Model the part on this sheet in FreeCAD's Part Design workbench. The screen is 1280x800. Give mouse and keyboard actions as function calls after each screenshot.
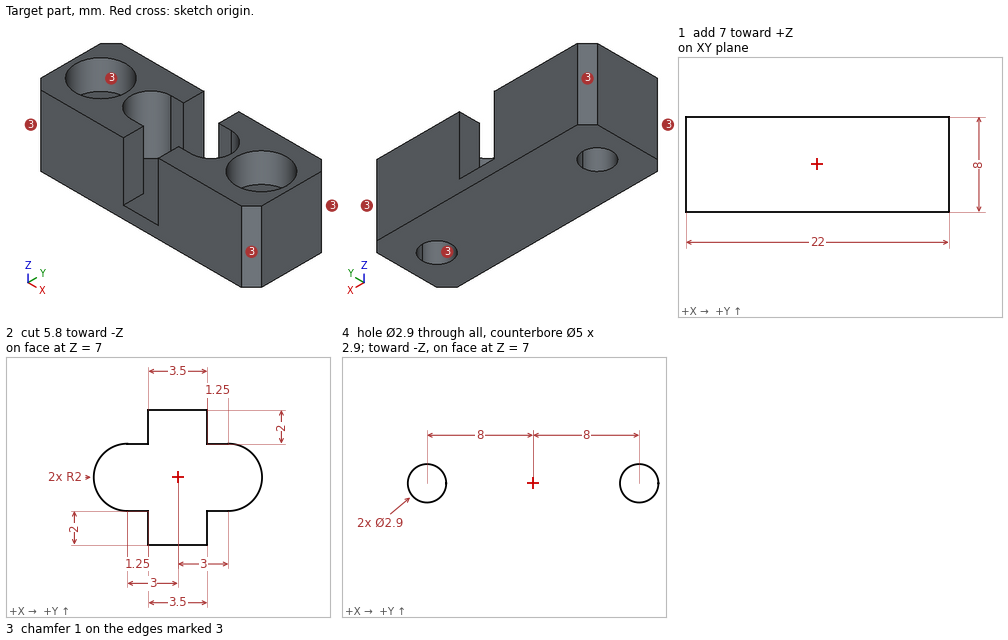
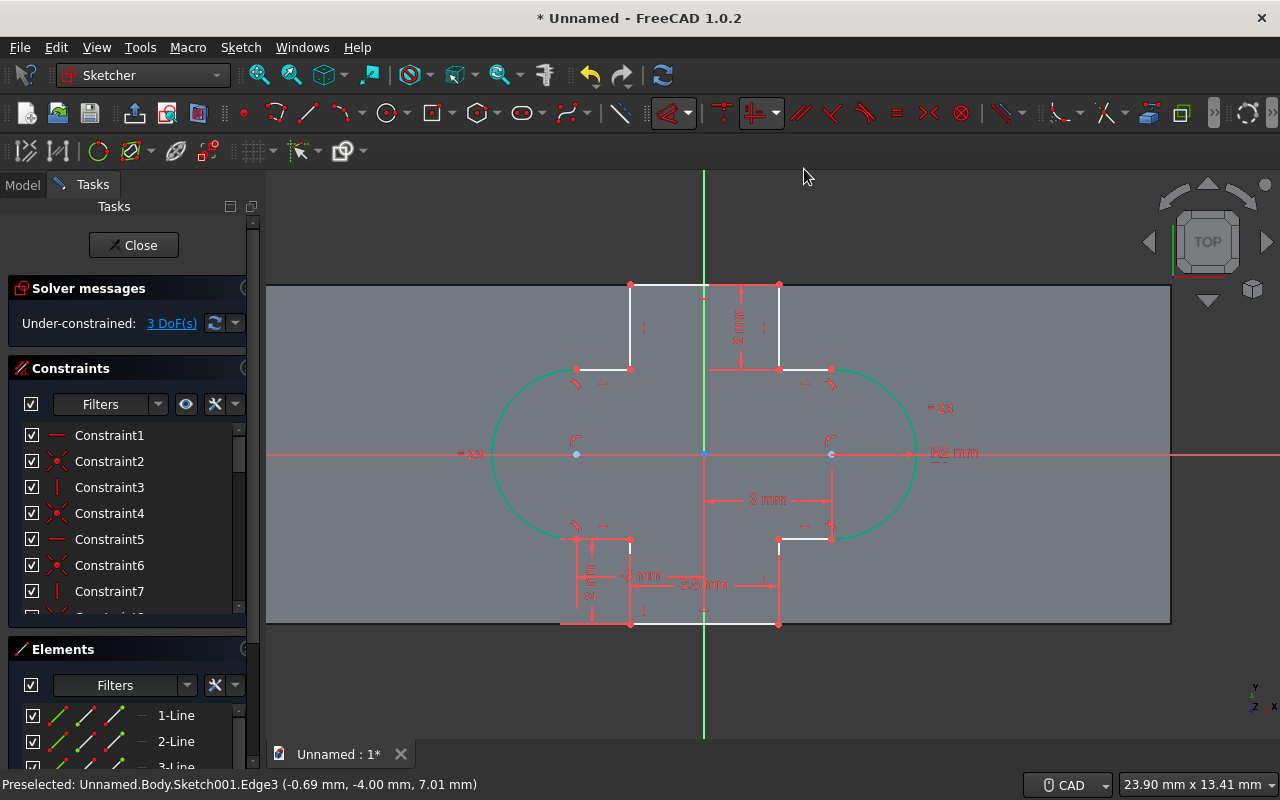
click(734, 285)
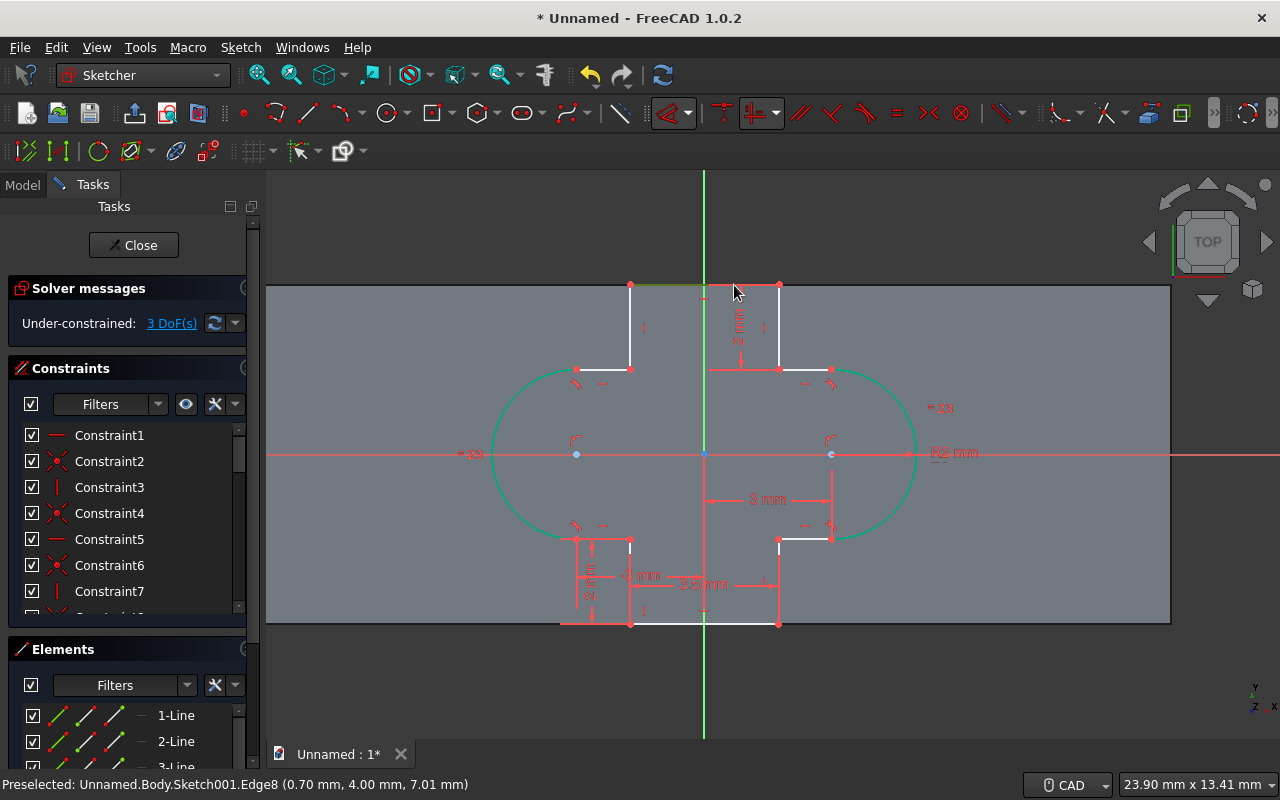
click(690, 114)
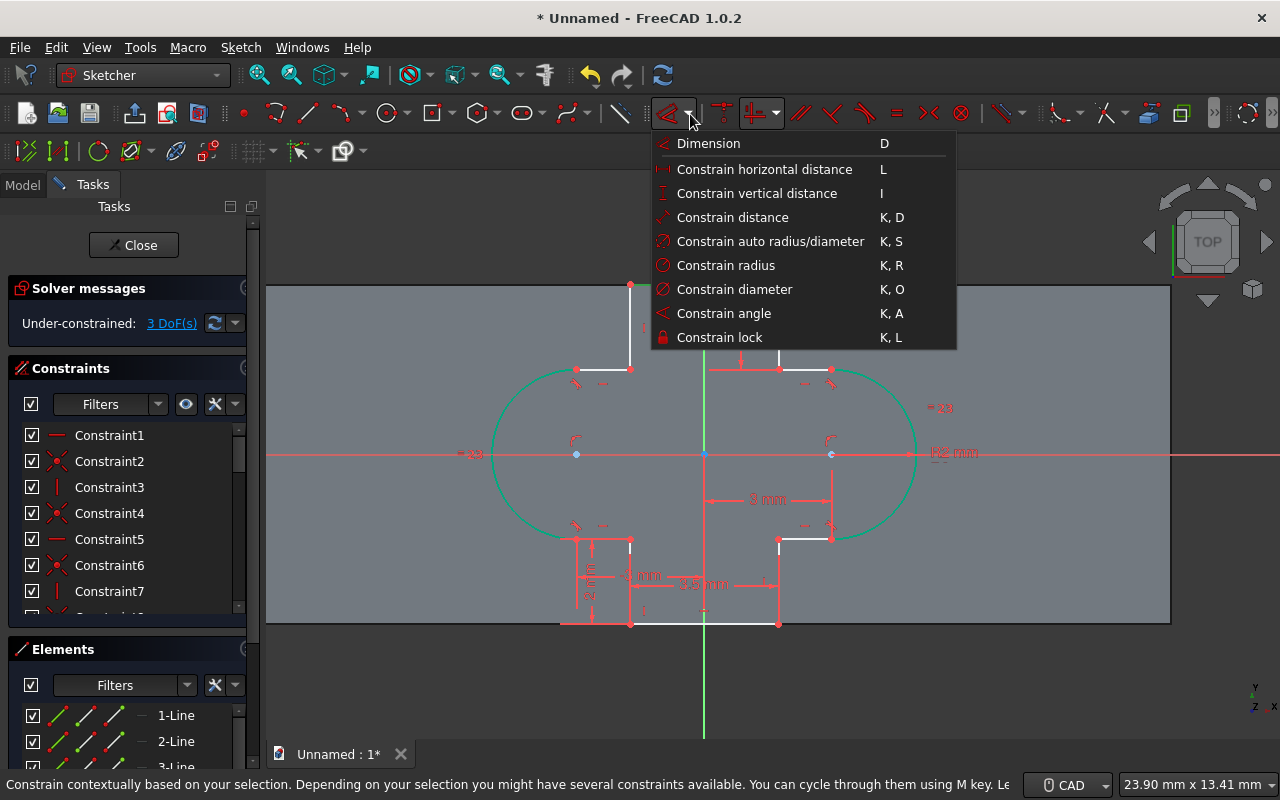
click(804, 169)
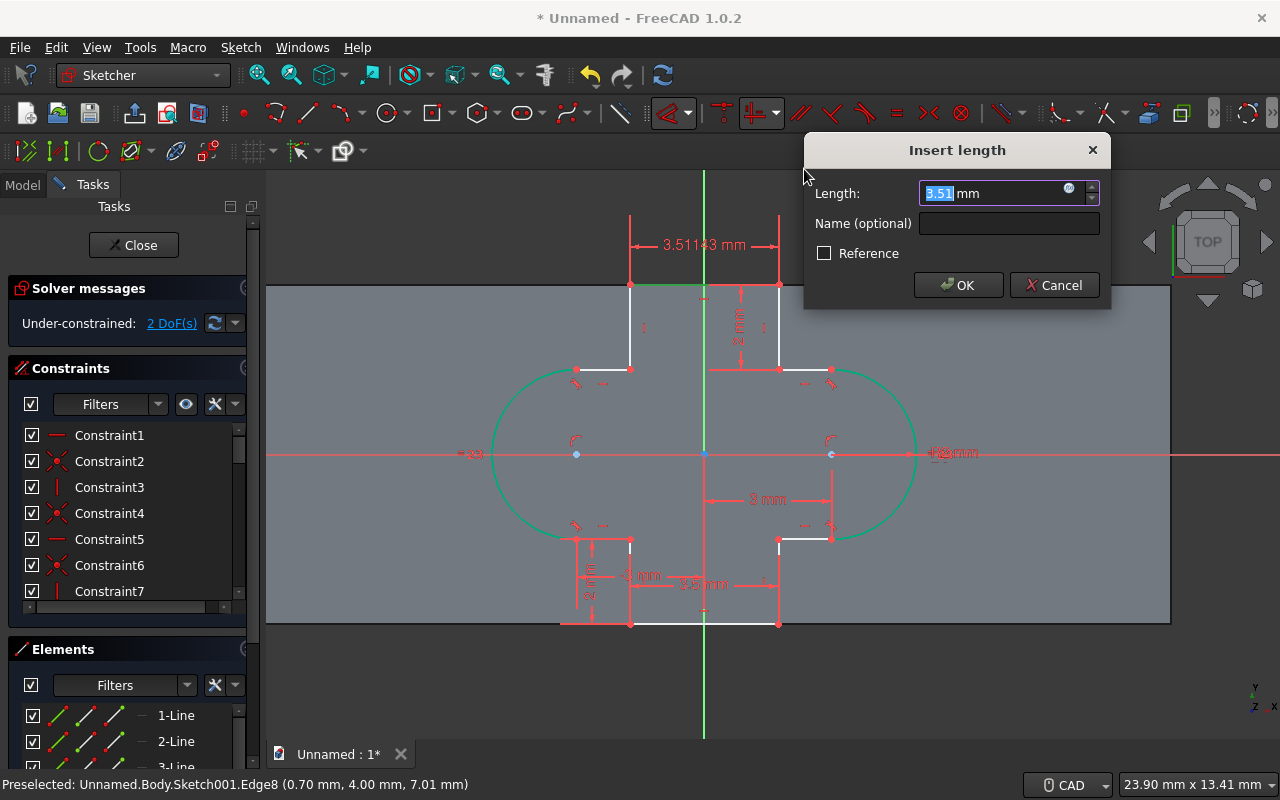
text(3.5)
key(Return)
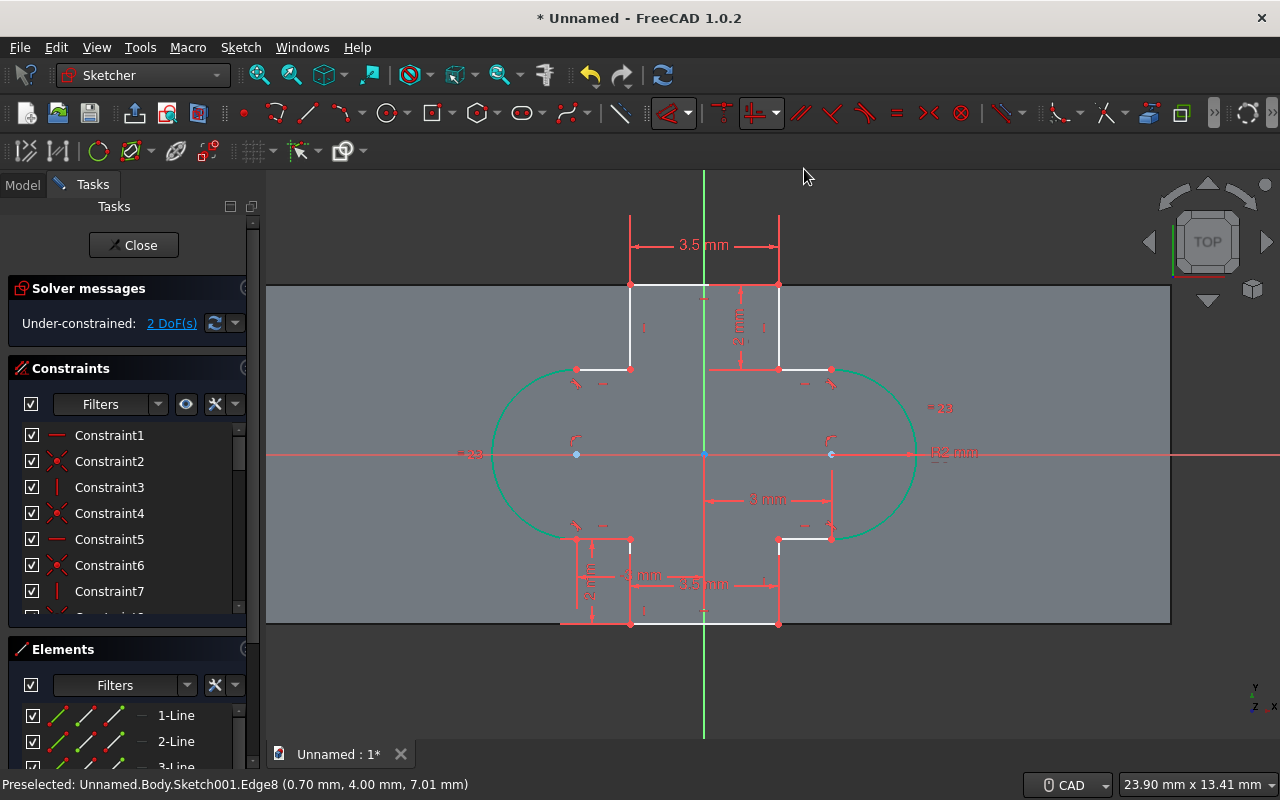
click(593, 539)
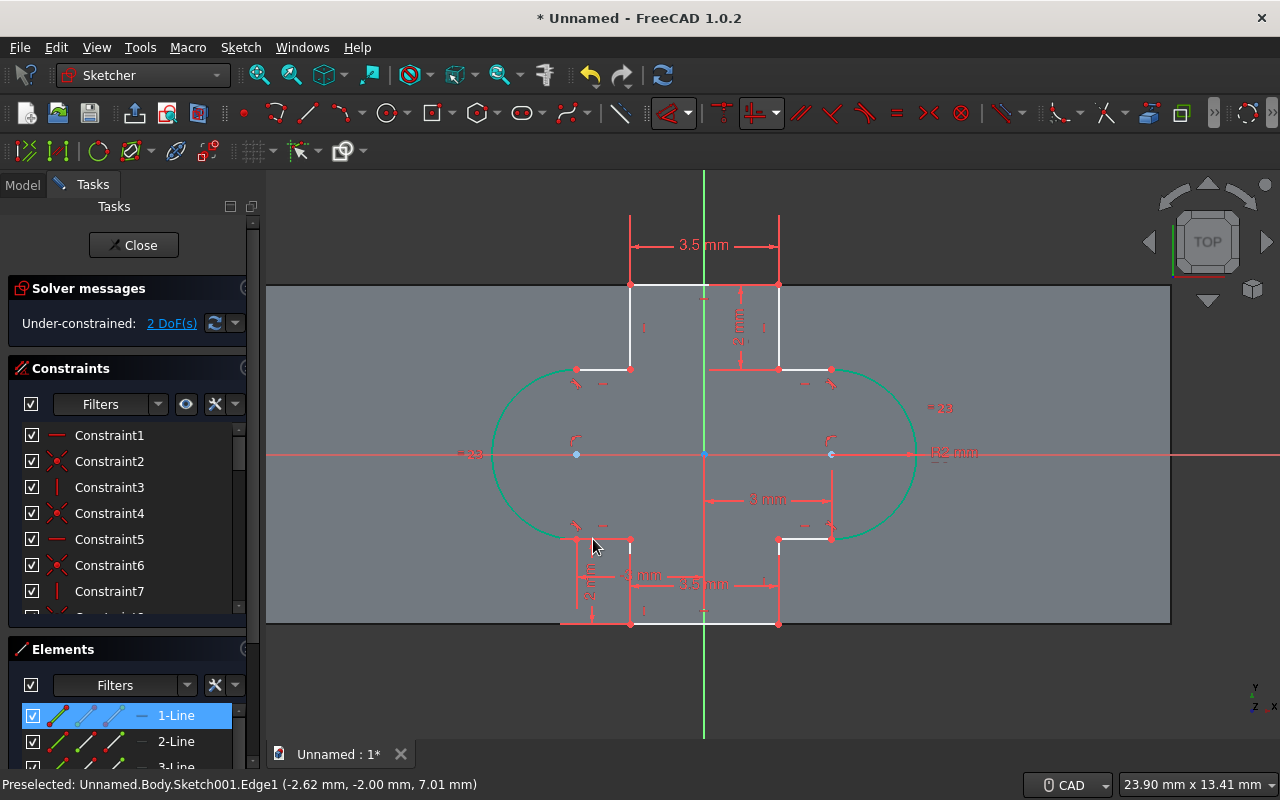
key(l)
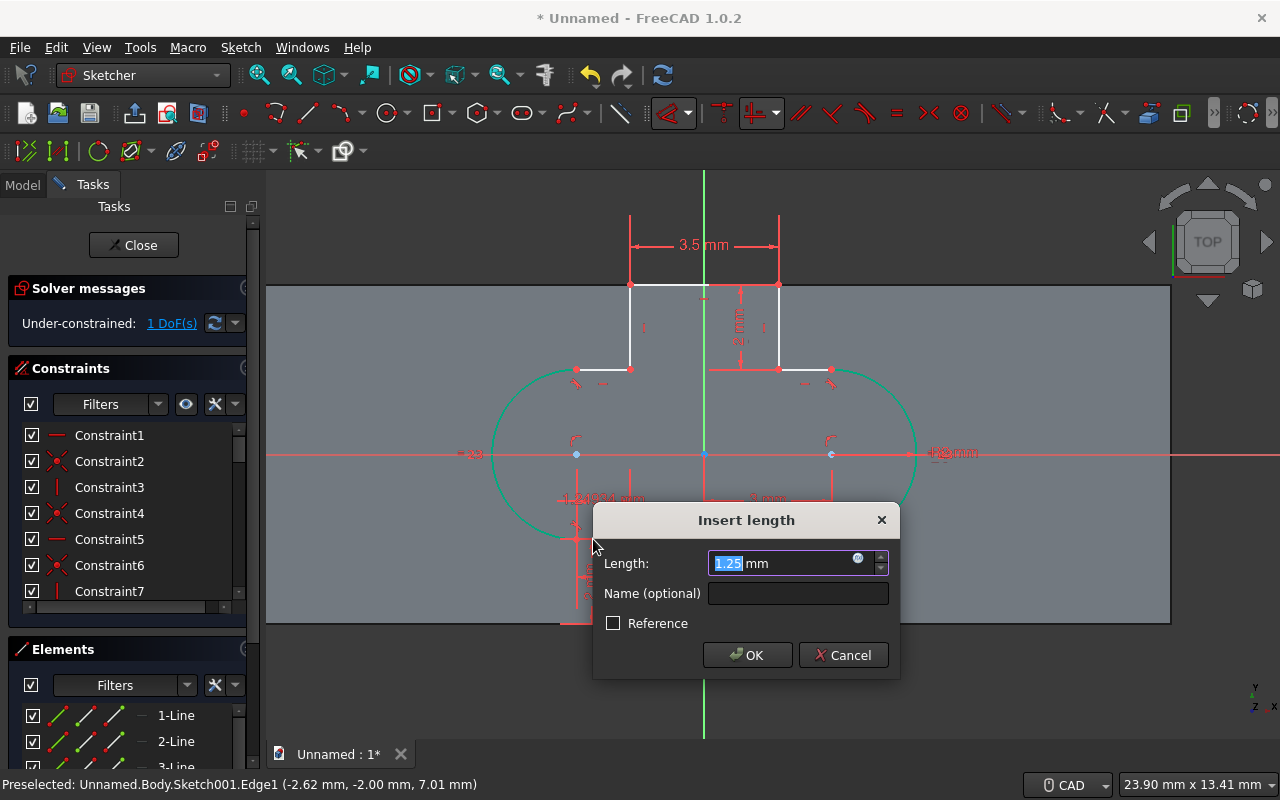
text(1.25)
key(Return)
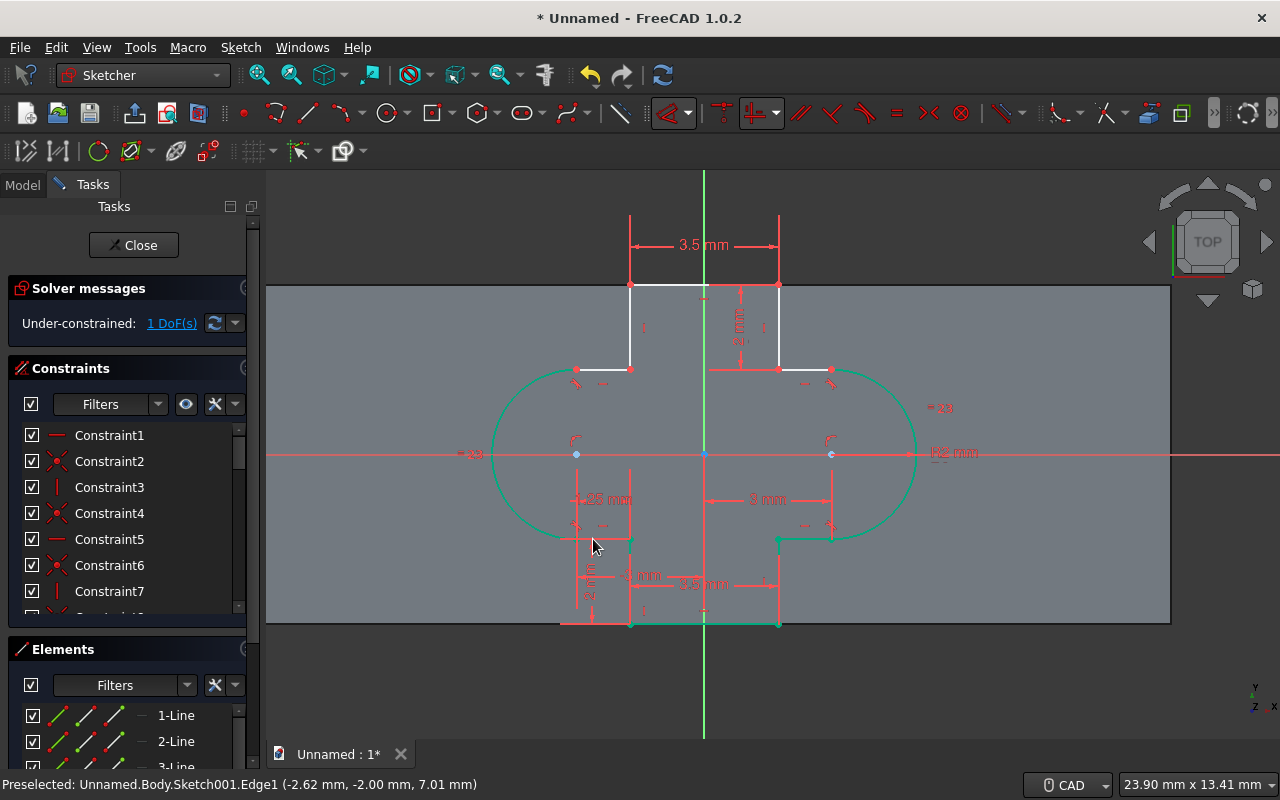
click(816, 370)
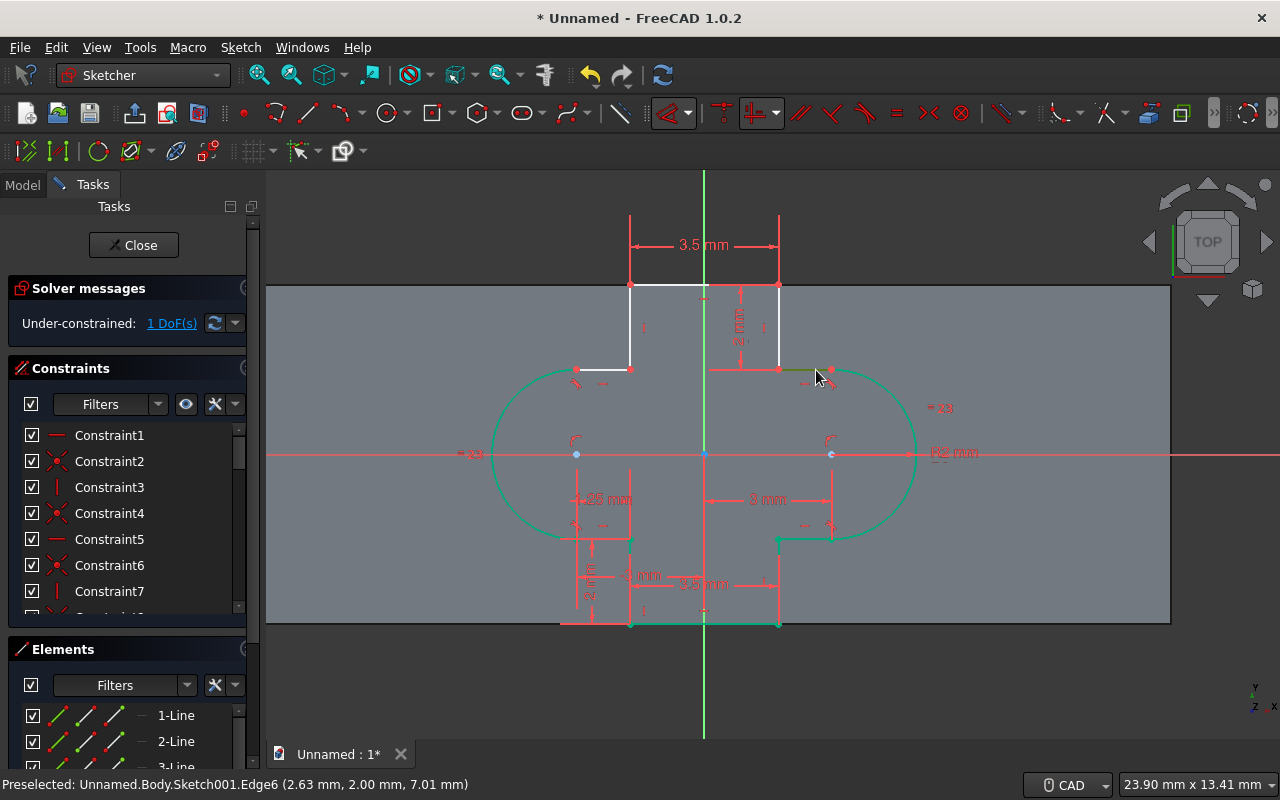
key(l)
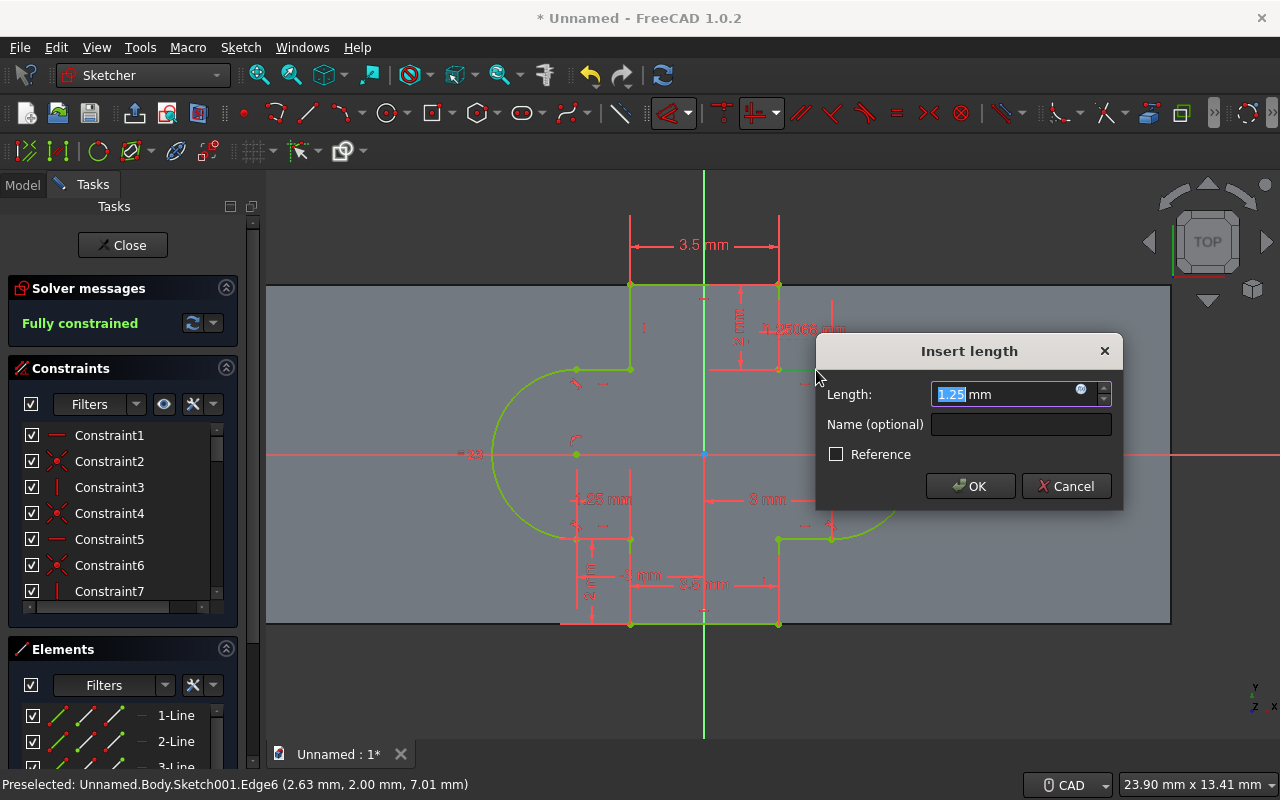
text(1.25)
key(Return)